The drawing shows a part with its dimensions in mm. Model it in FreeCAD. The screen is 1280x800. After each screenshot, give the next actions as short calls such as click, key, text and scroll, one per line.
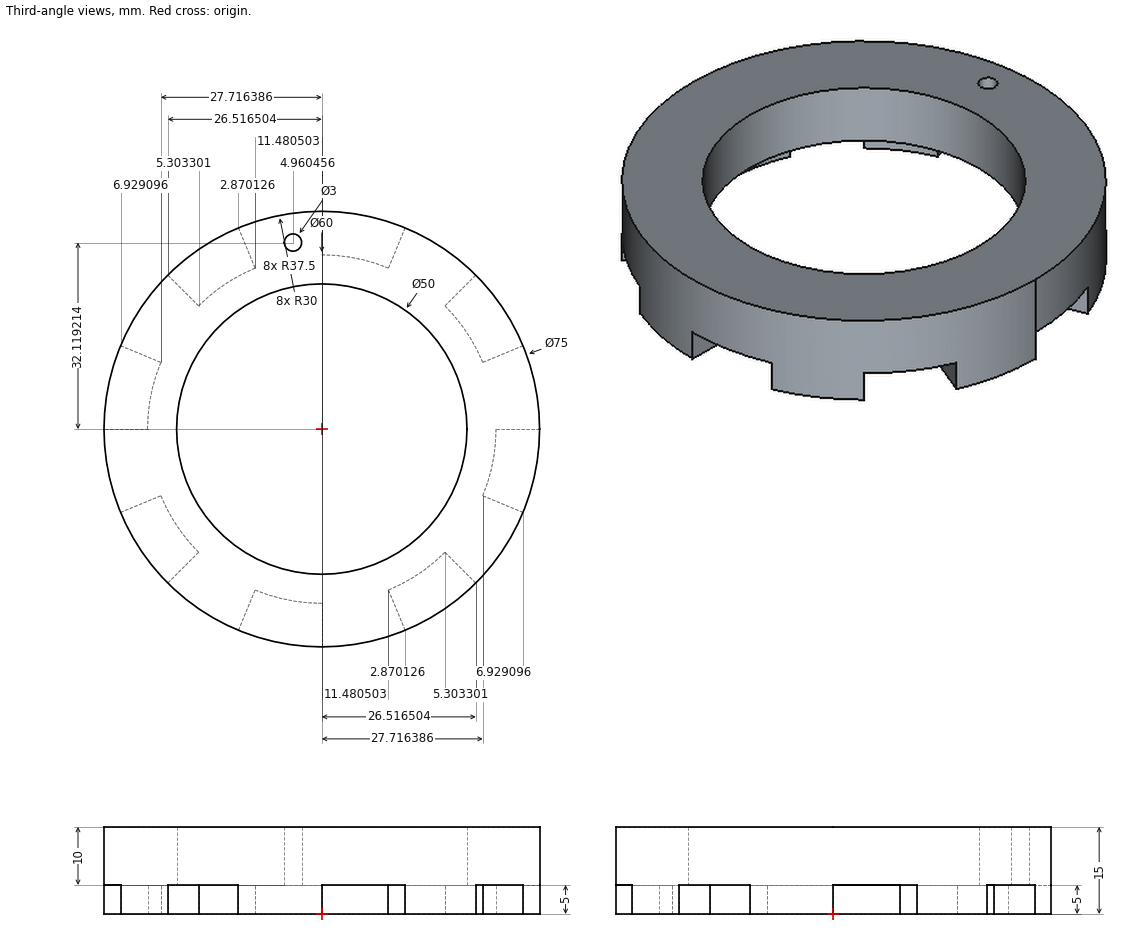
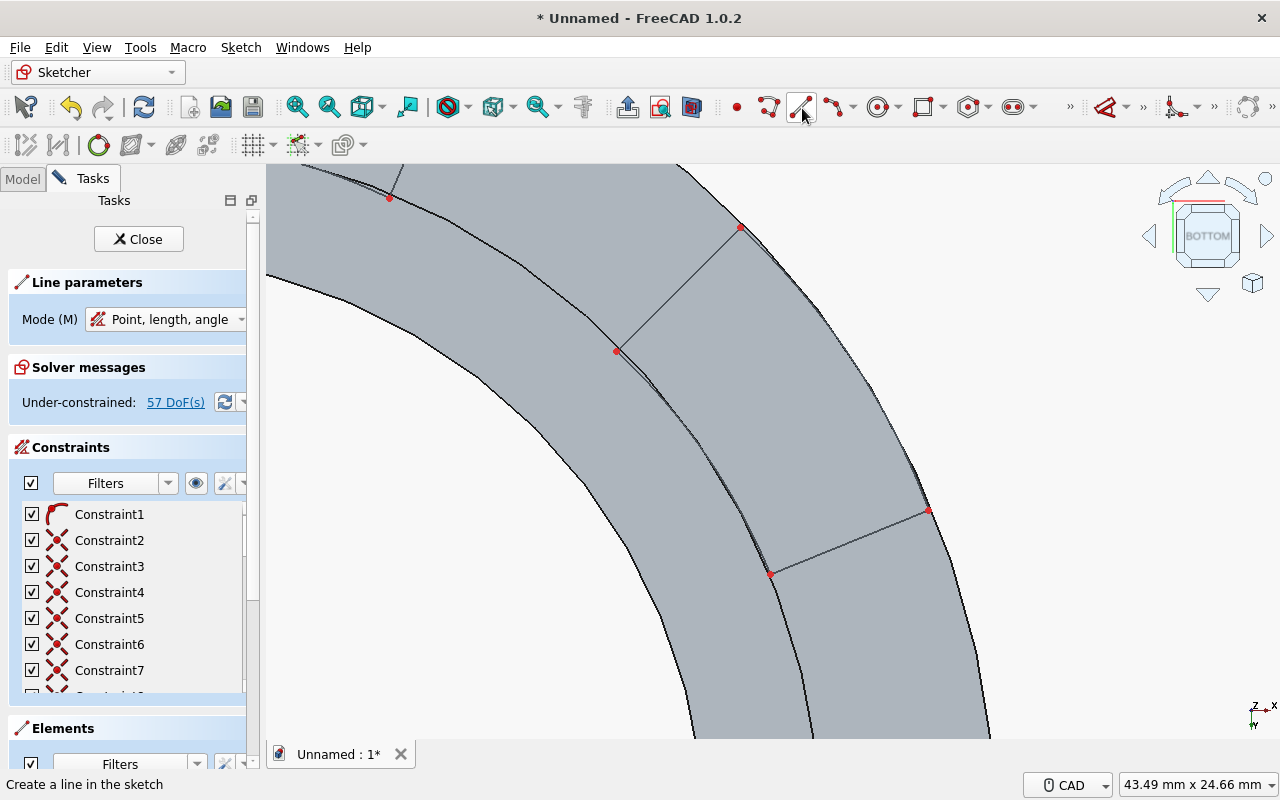
scroll(852, 353, down, 8)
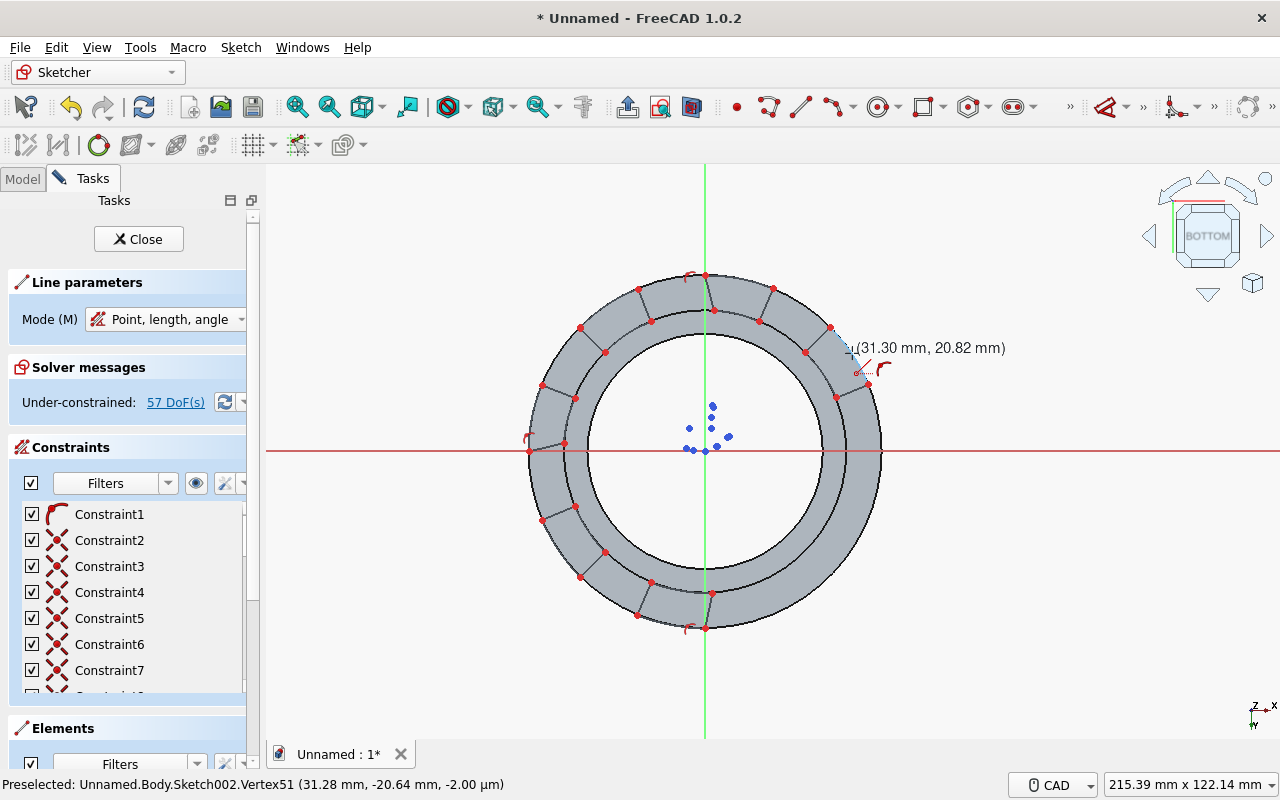
click(882, 451)
click(846, 442)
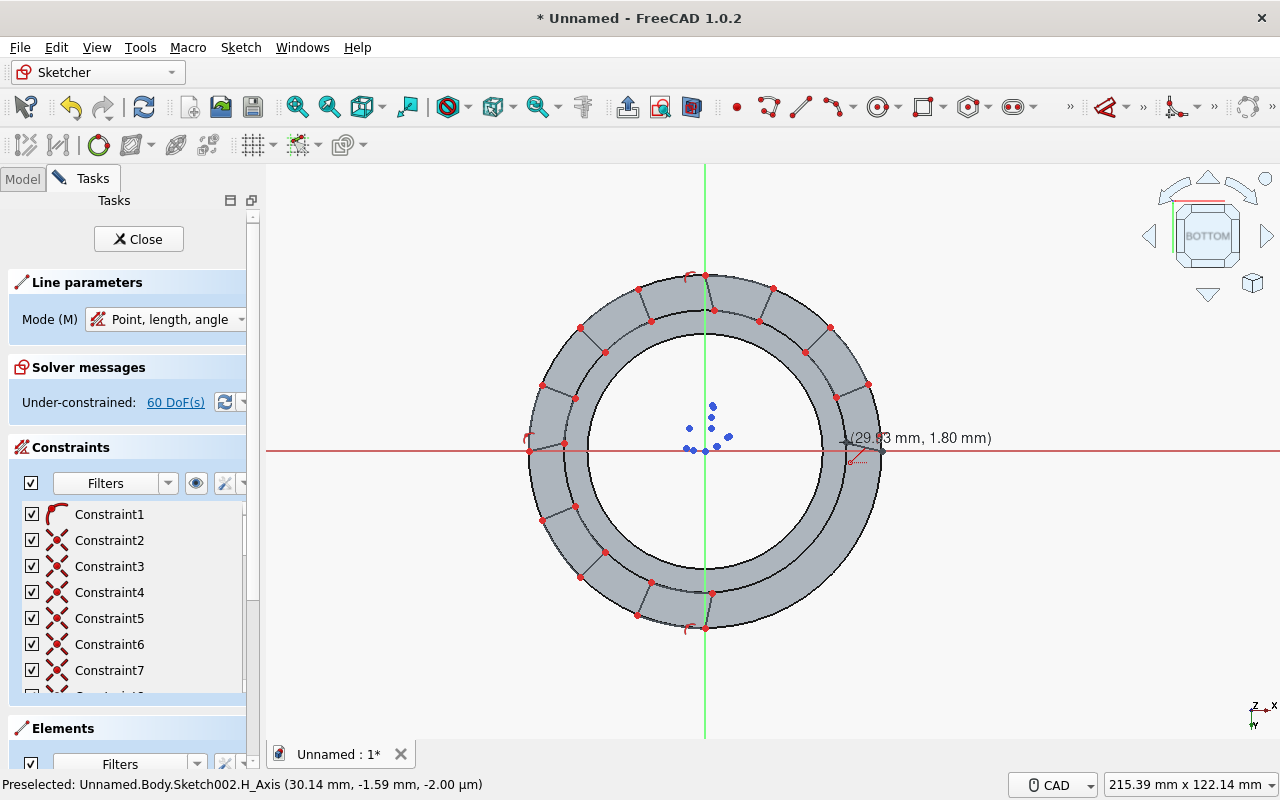
click(836, 506)
click(868, 519)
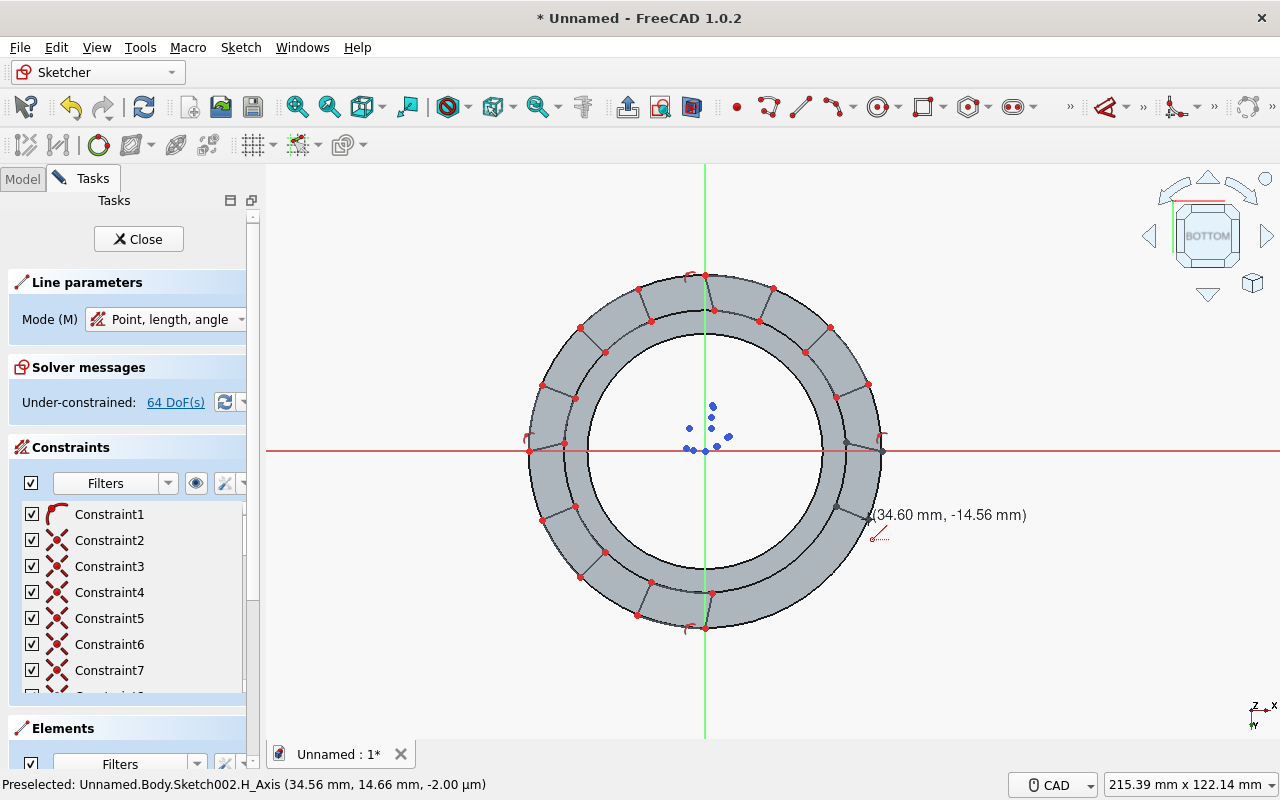
key(g)
key(3)
key(a)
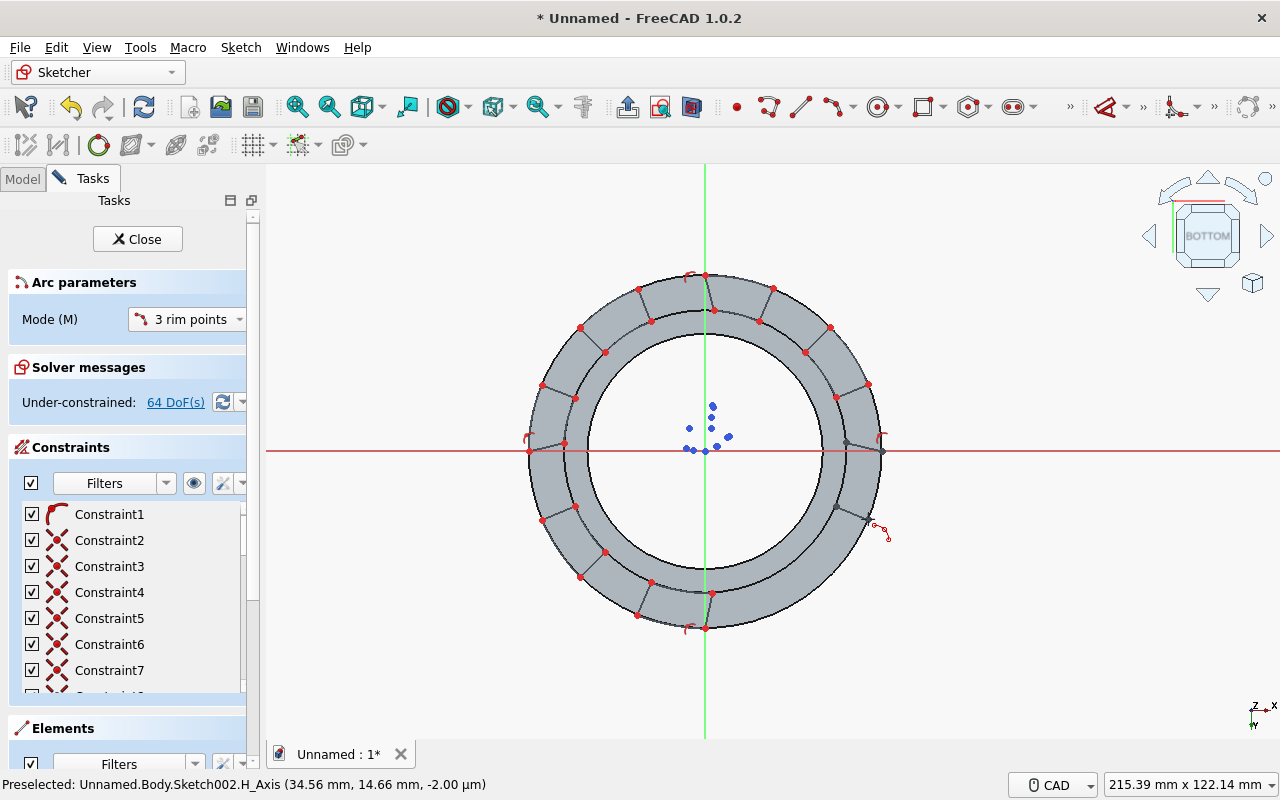
click(846, 443)
click(836, 507)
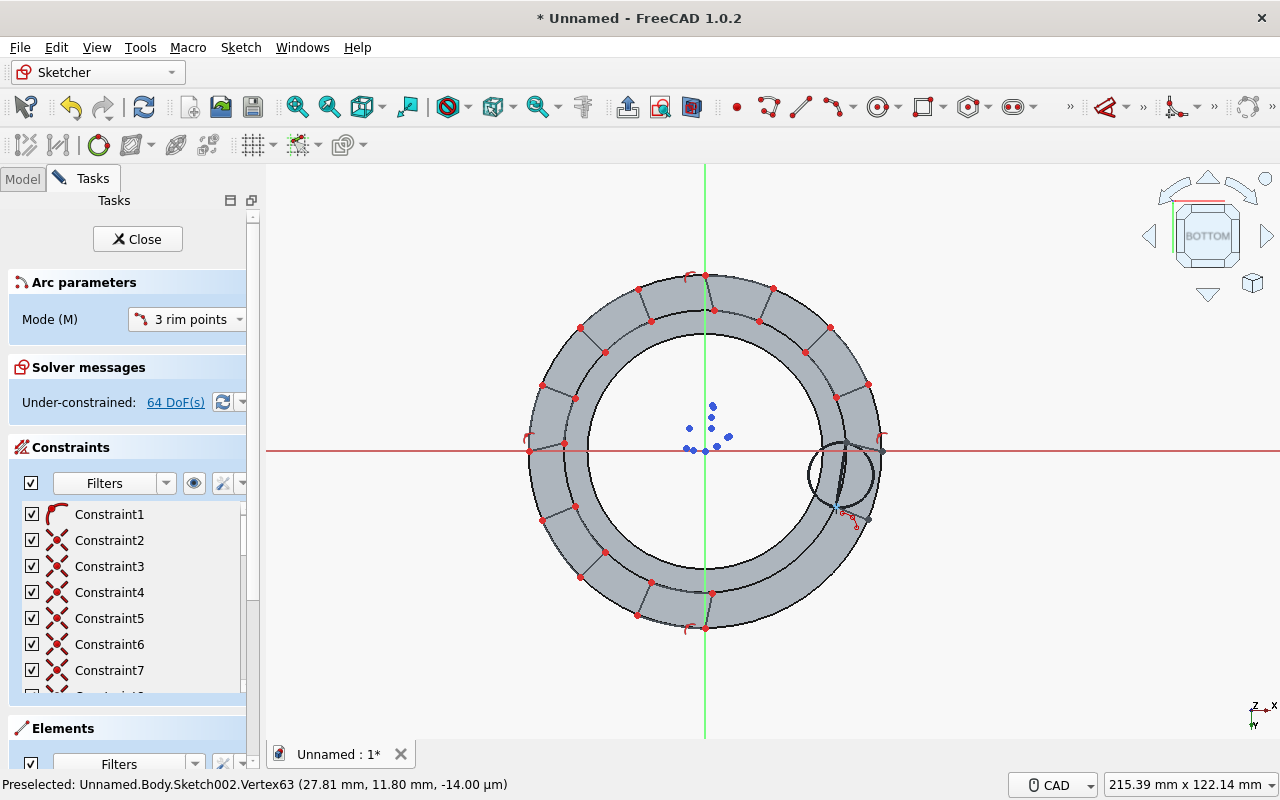
scroll(844, 479, up, 9)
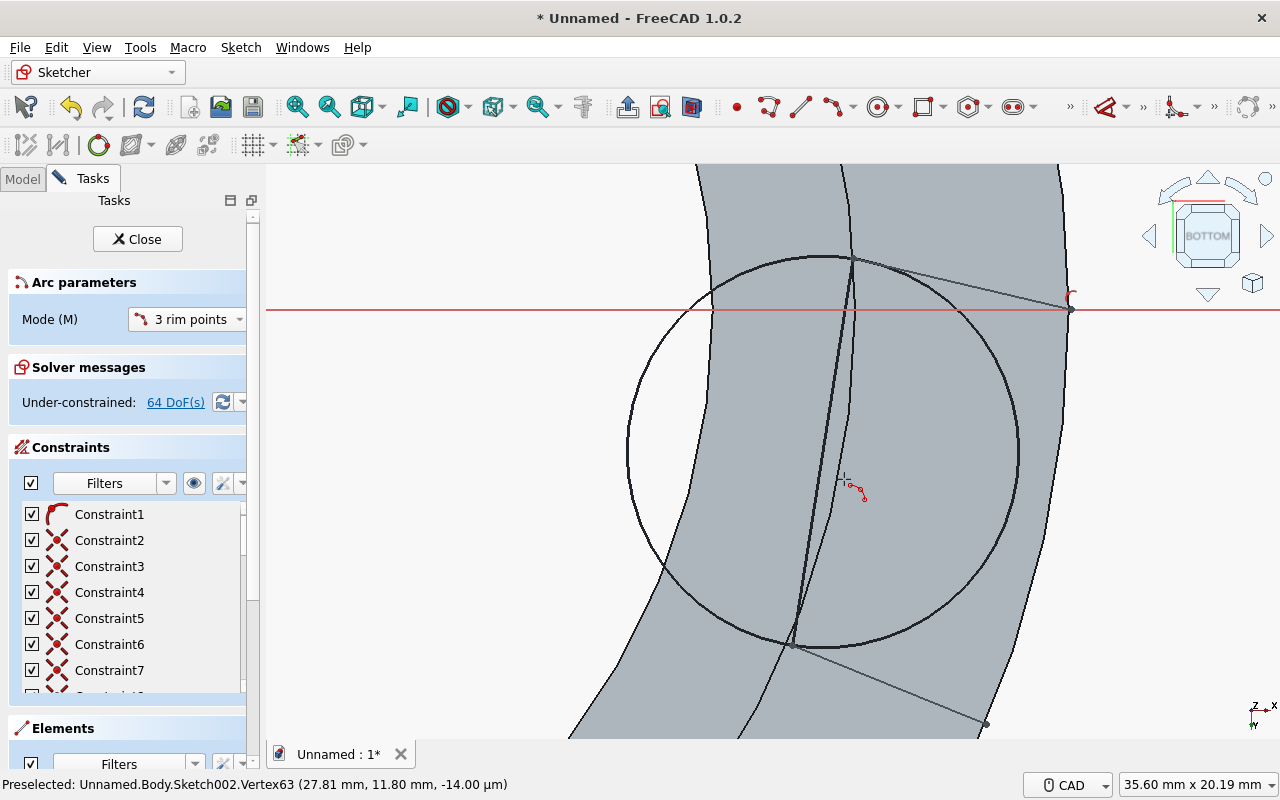
click(839, 476)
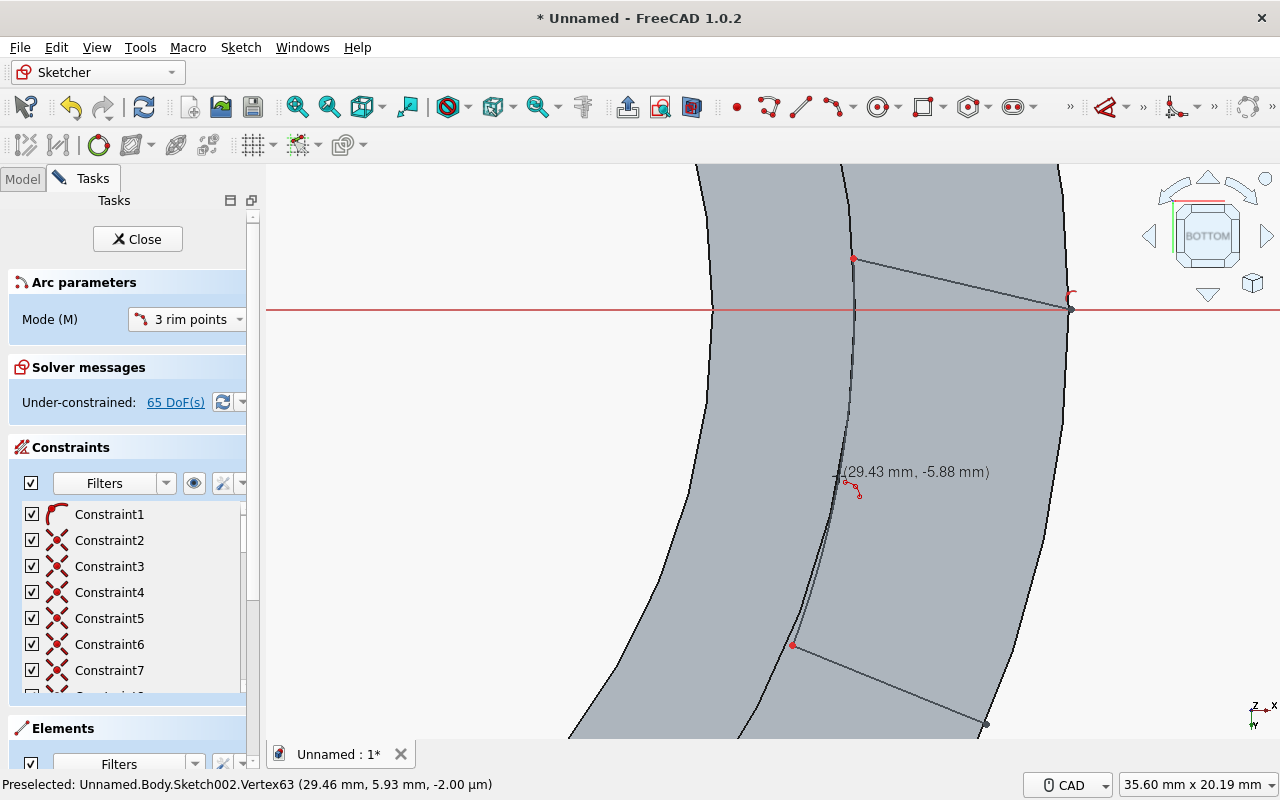
scroll(844, 480, down, 9)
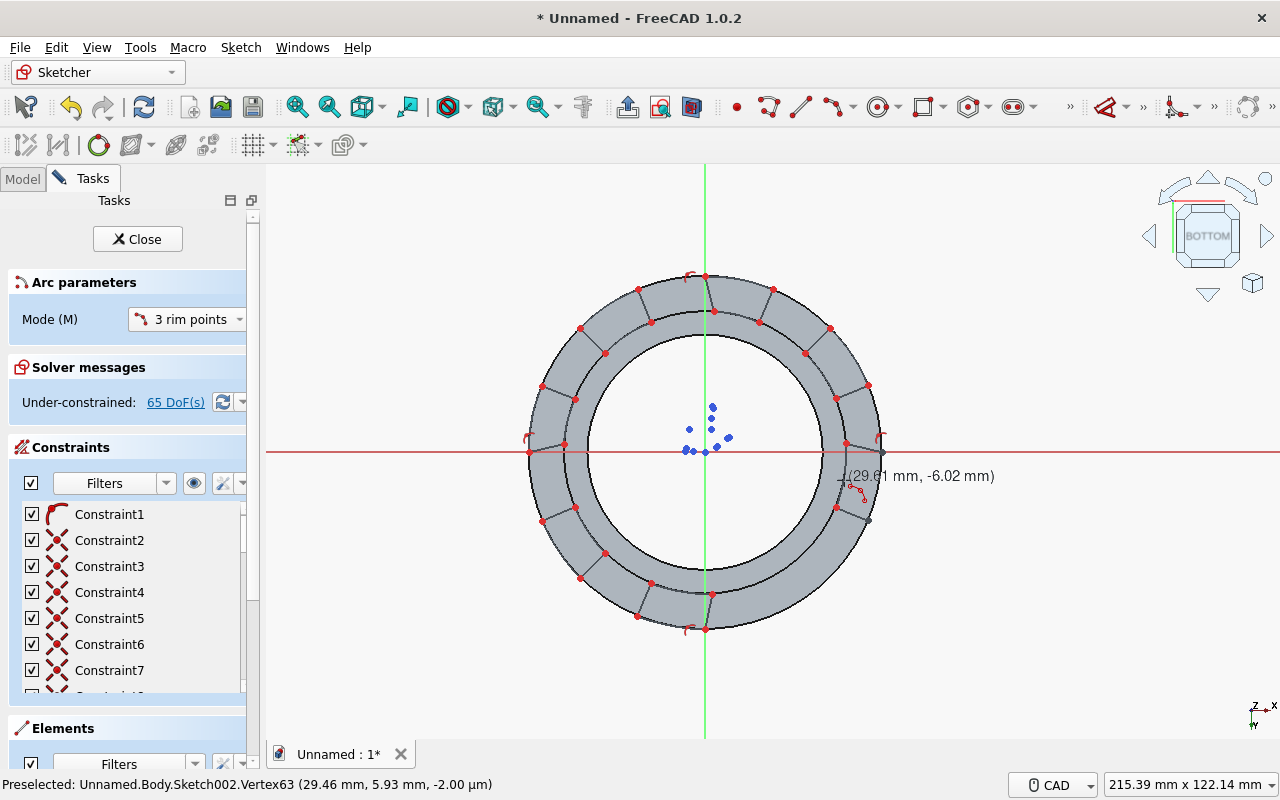
click(868, 521)
click(882, 452)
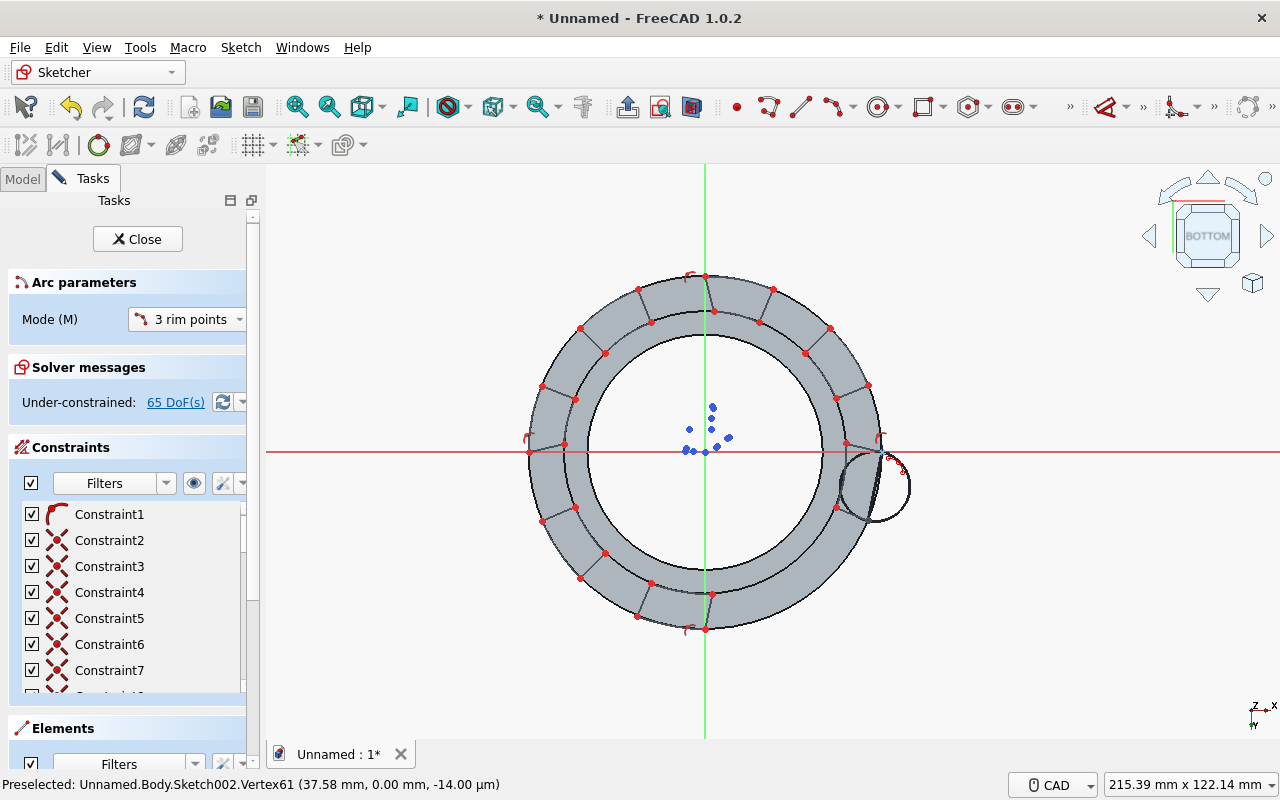
scroll(878, 487, up, 8)